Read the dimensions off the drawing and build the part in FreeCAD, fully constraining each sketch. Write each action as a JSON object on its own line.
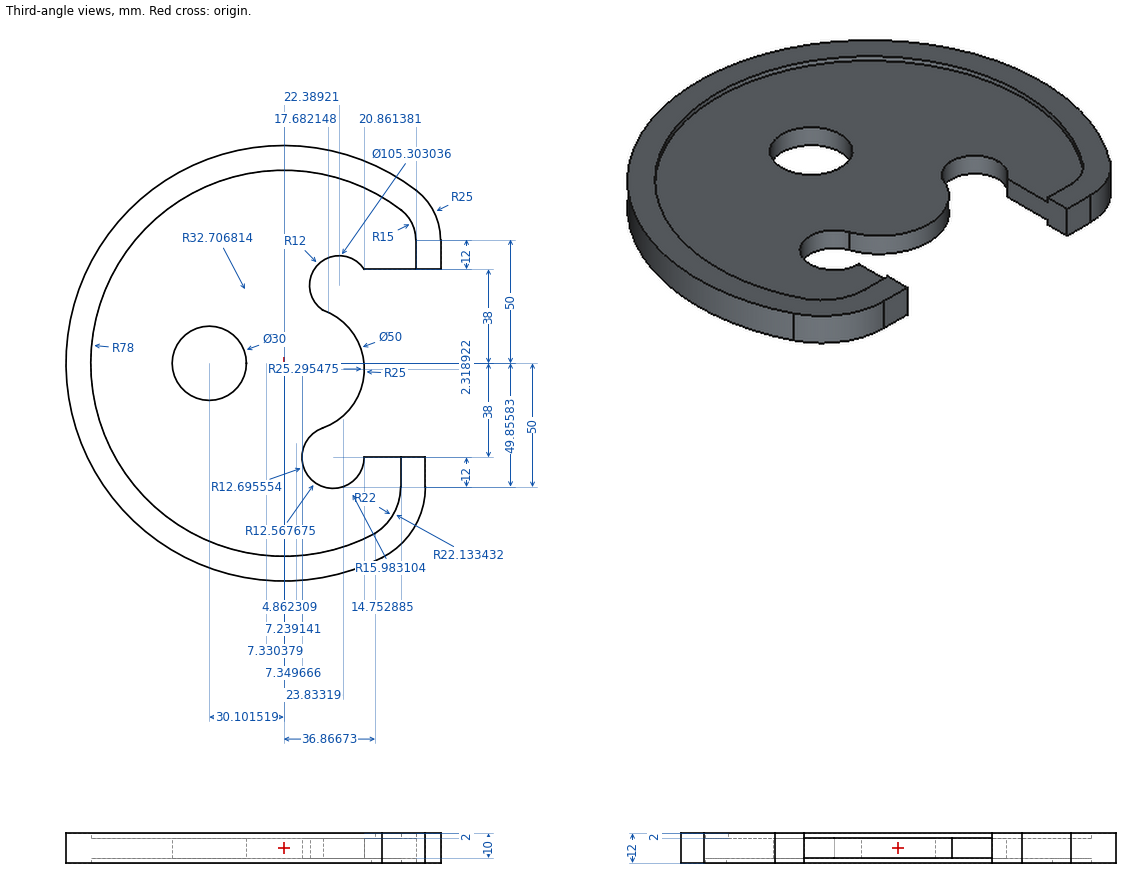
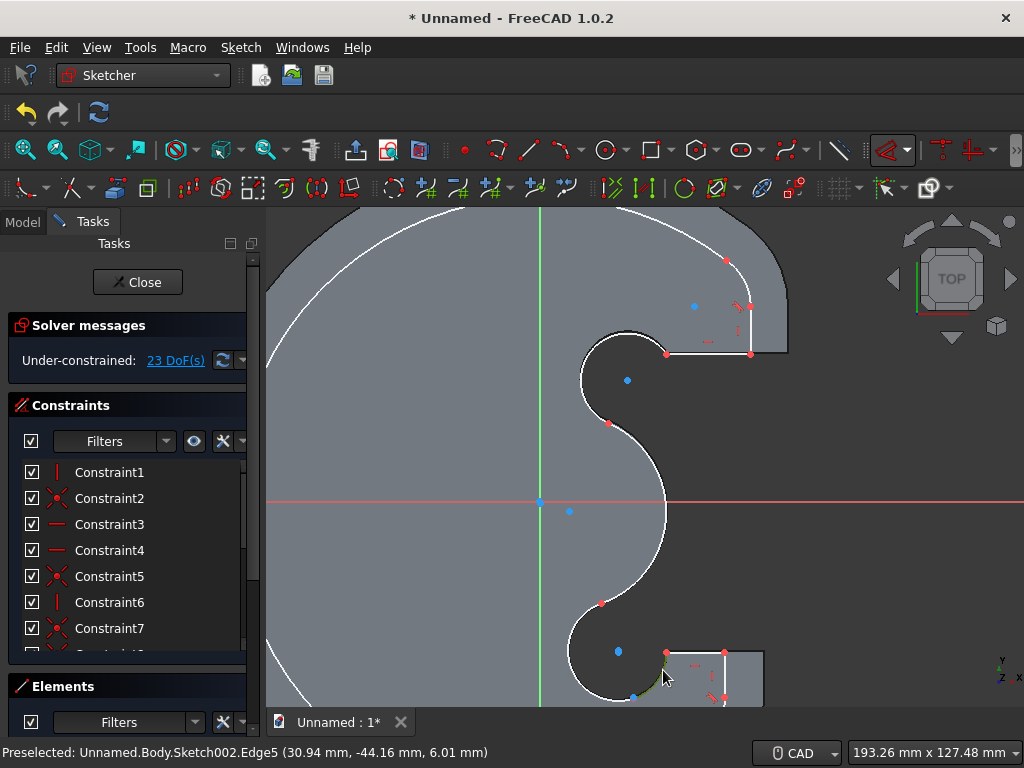
{"action": "left_click", "coordinate": [570, 636]}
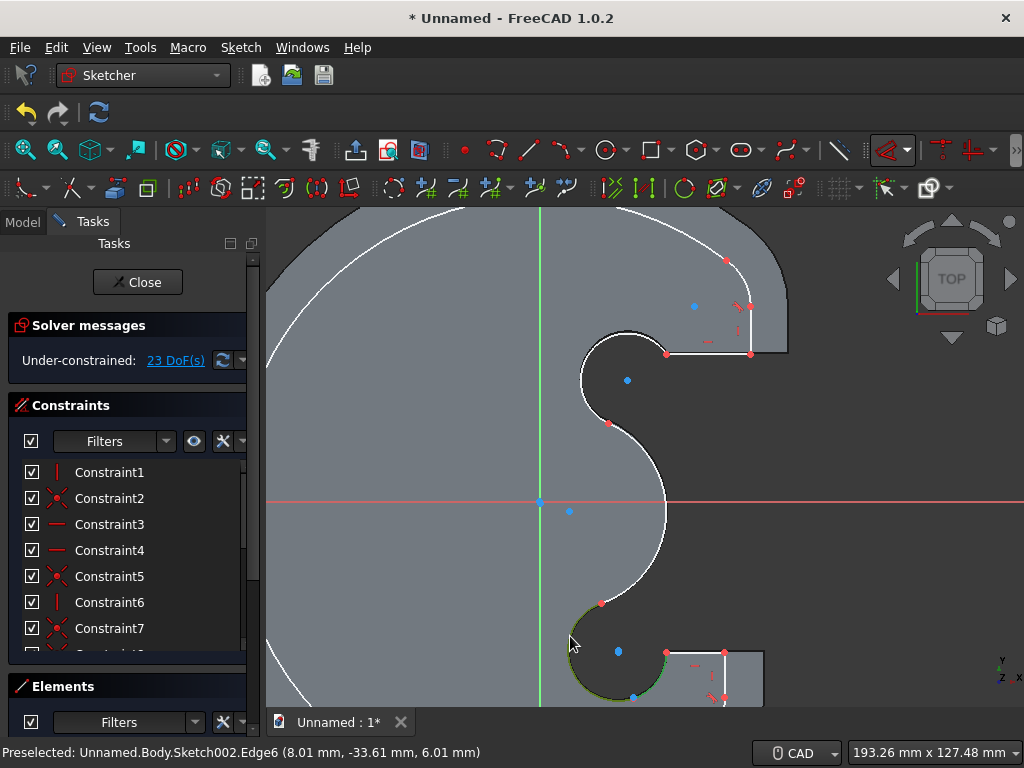
{"action": "key", "text": "t"}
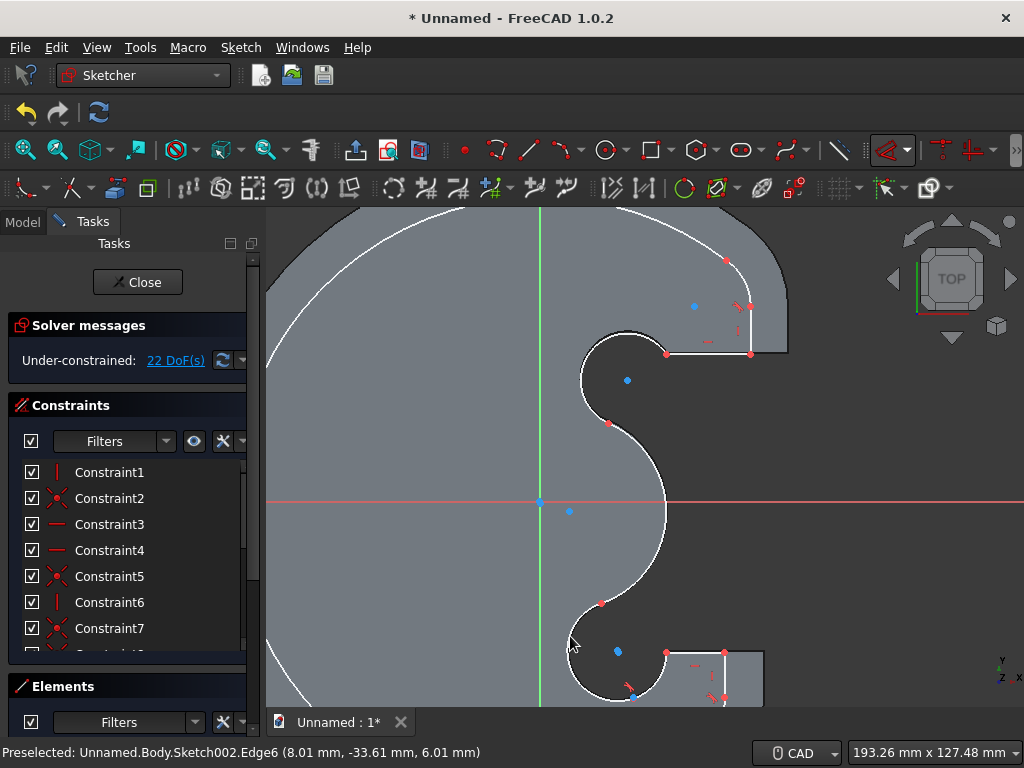
{"action": "left_click", "coordinate": [570, 636]}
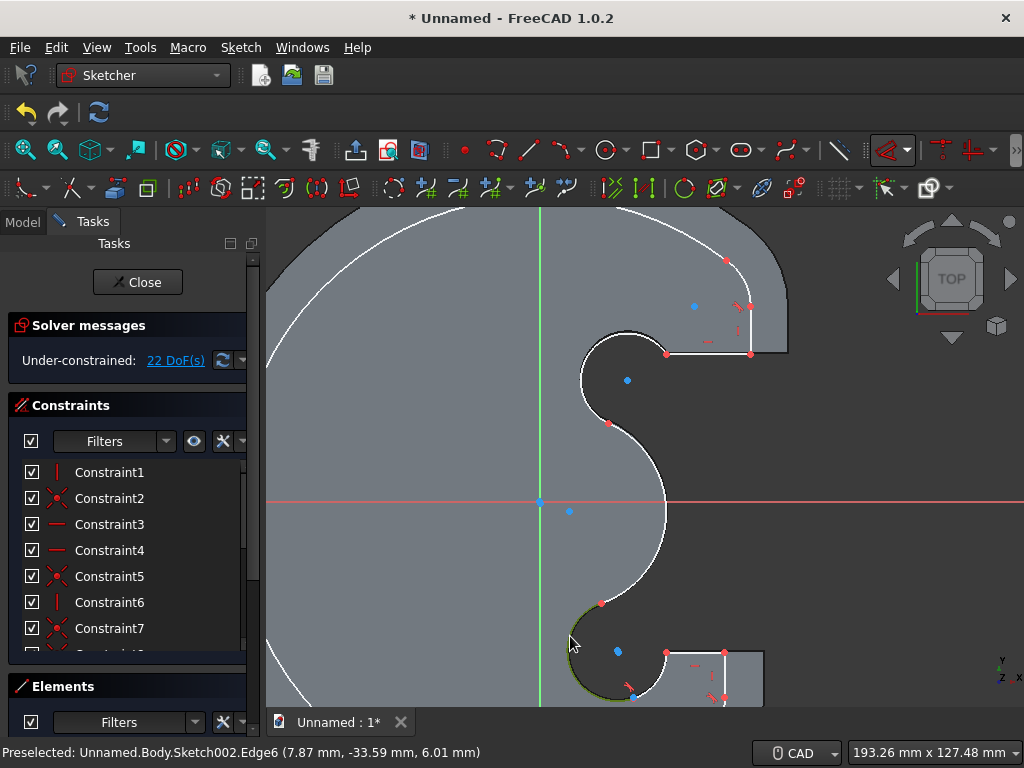
{"action": "left_click", "coordinate": [653, 560]}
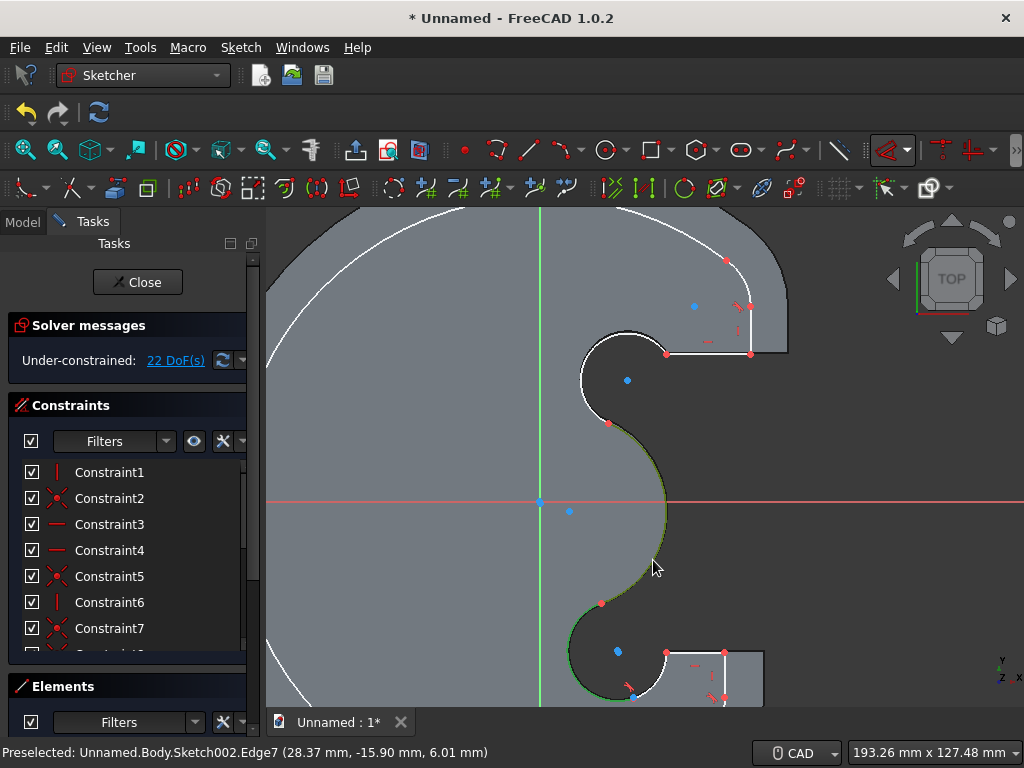
{"action": "key", "text": "t"}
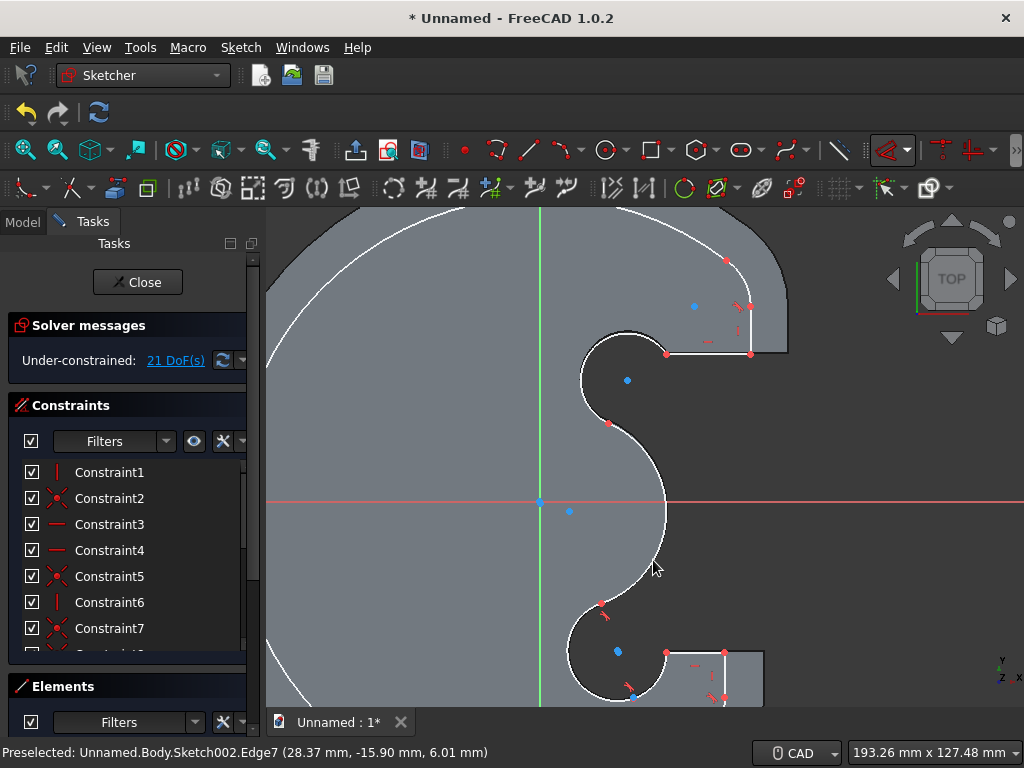
{"action": "left_click", "coordinate": [748, 291]}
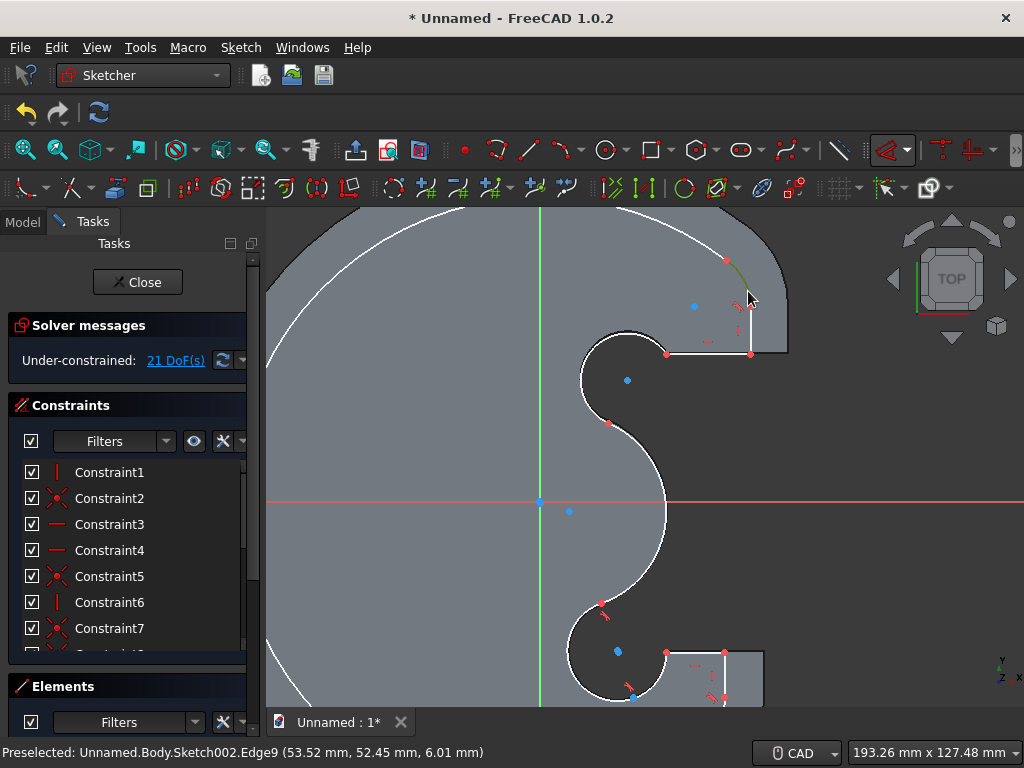
{"action": "left_click", "coordinate": [359, 256]}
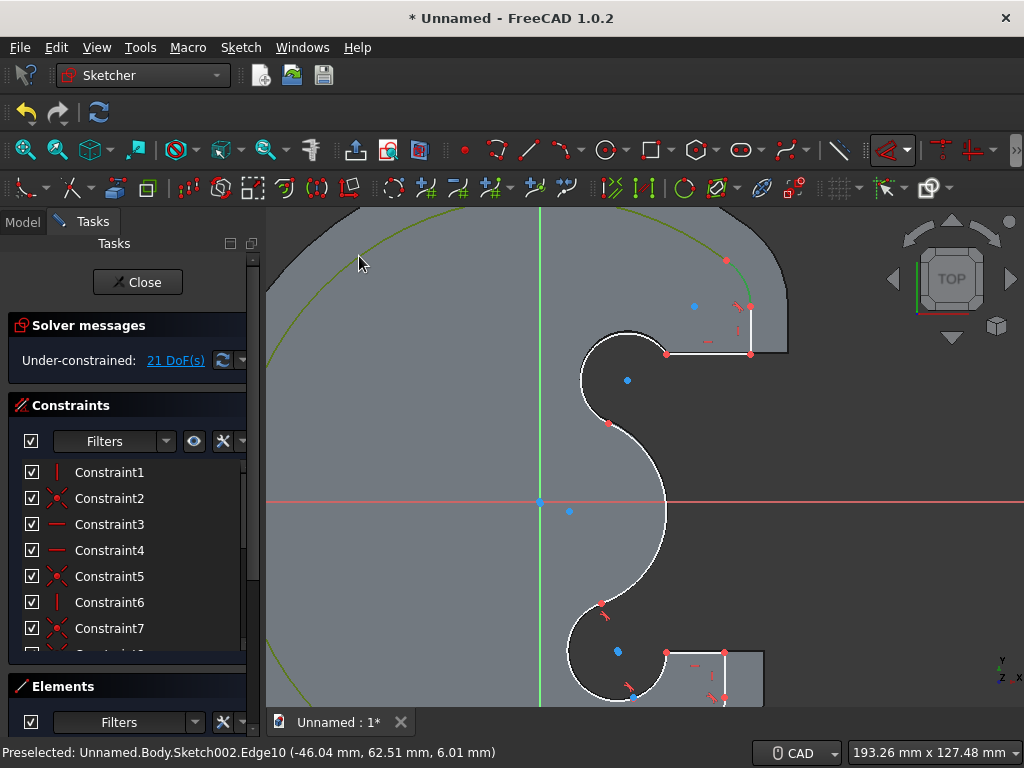
{"action": "key", "text": "t"}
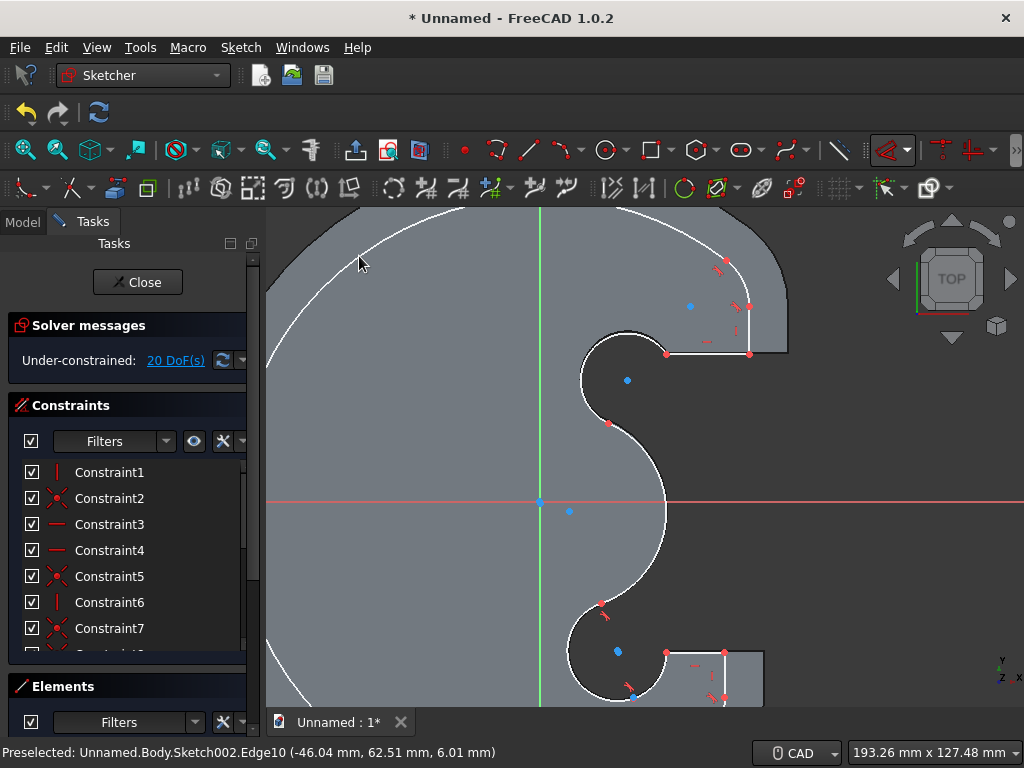
{"action": "left_click_drag", "start_coordinate": [530, 492], "coordinate": [550, 513]}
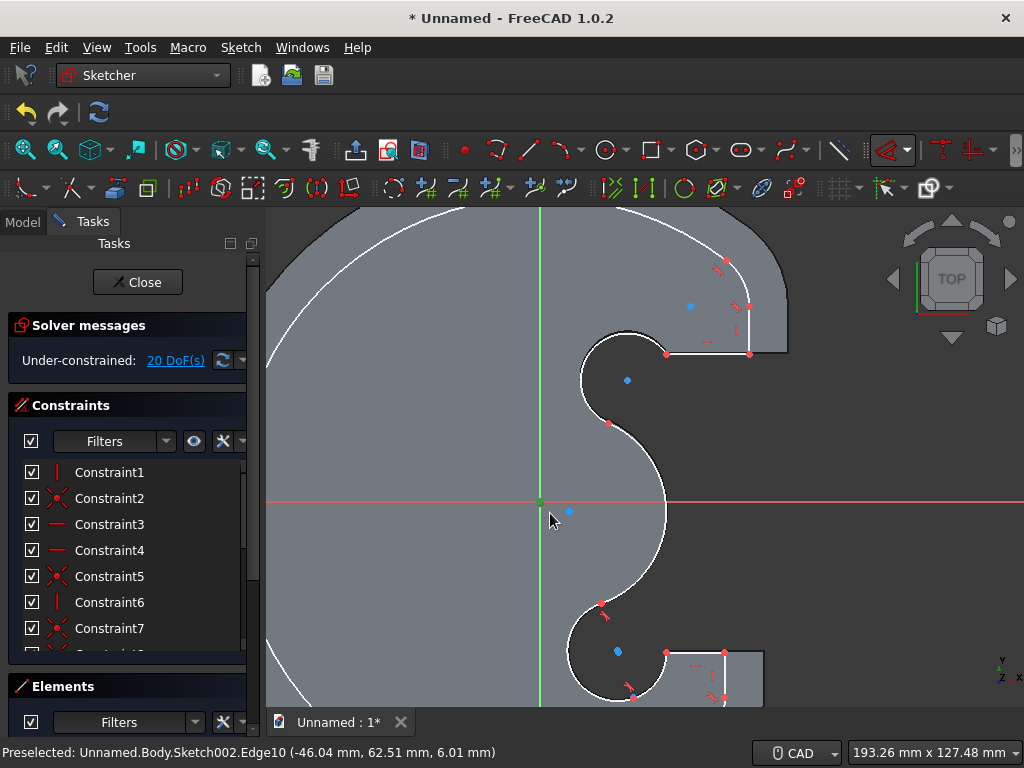
{"action": "key", "text": "c"}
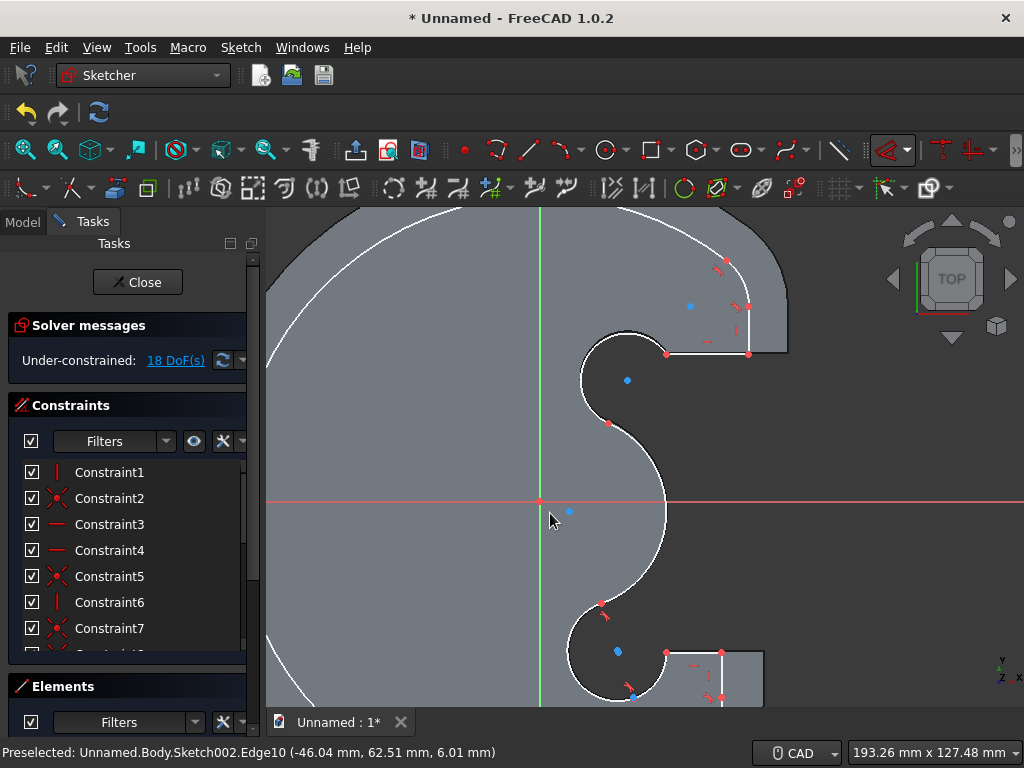
{"action": "left_click", "coordinate": [663, 670]}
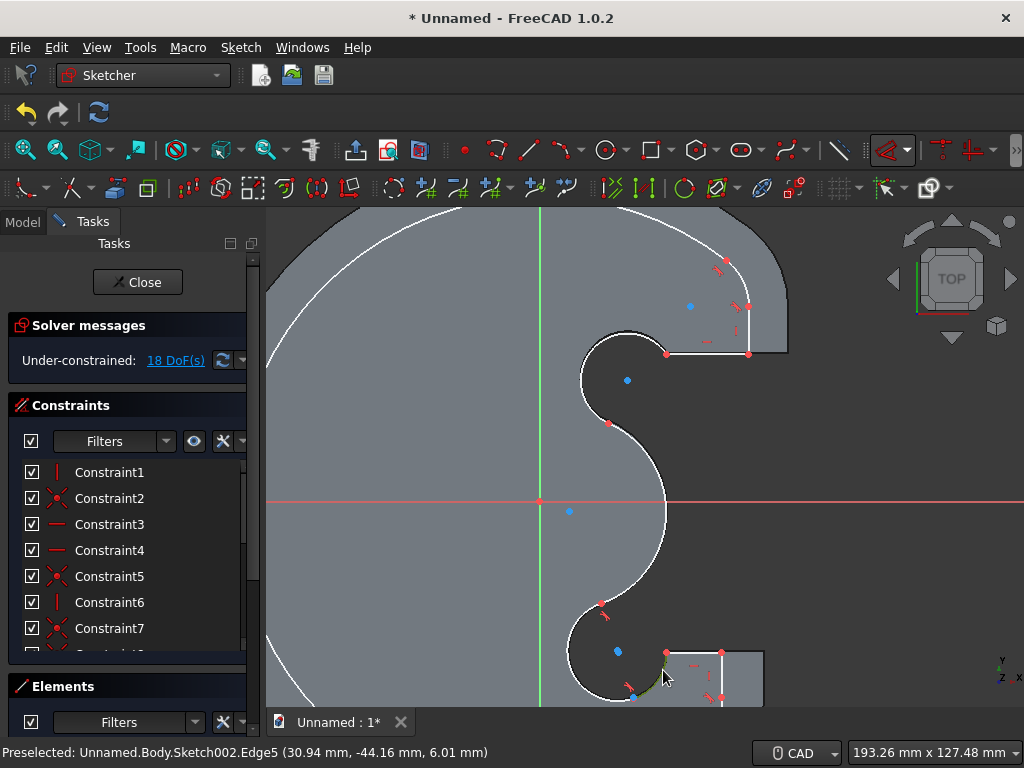
{"action": "key", "text": "k r"}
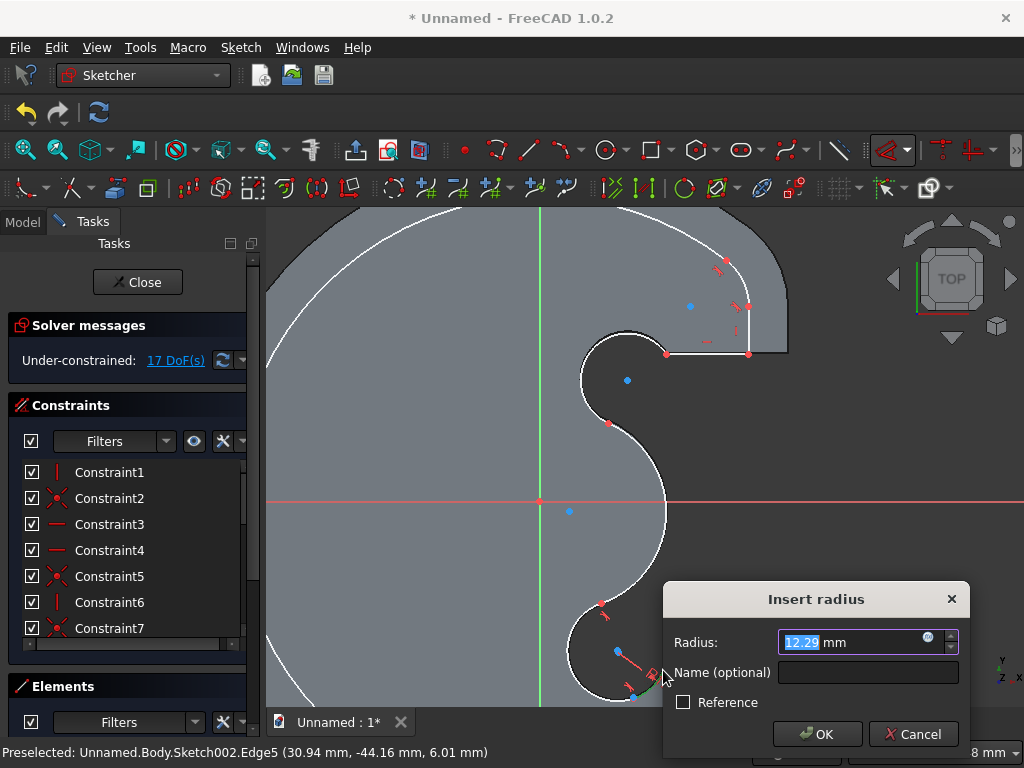
{"action": "type", "text": "12.567675"}
{"action": "key", "text": "Return"}